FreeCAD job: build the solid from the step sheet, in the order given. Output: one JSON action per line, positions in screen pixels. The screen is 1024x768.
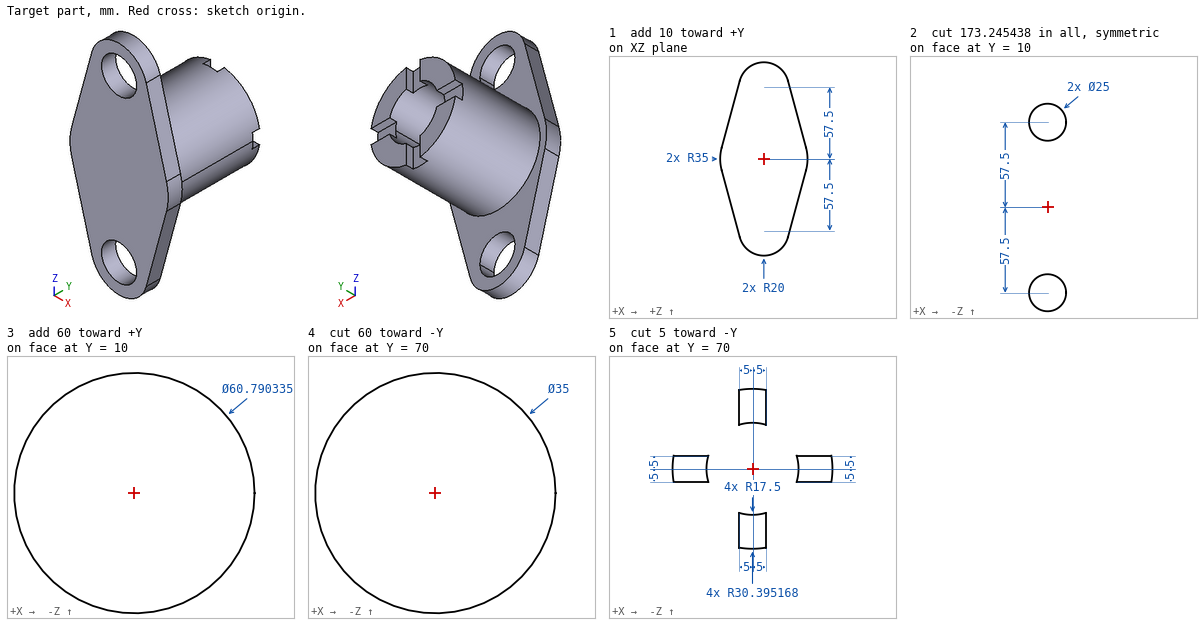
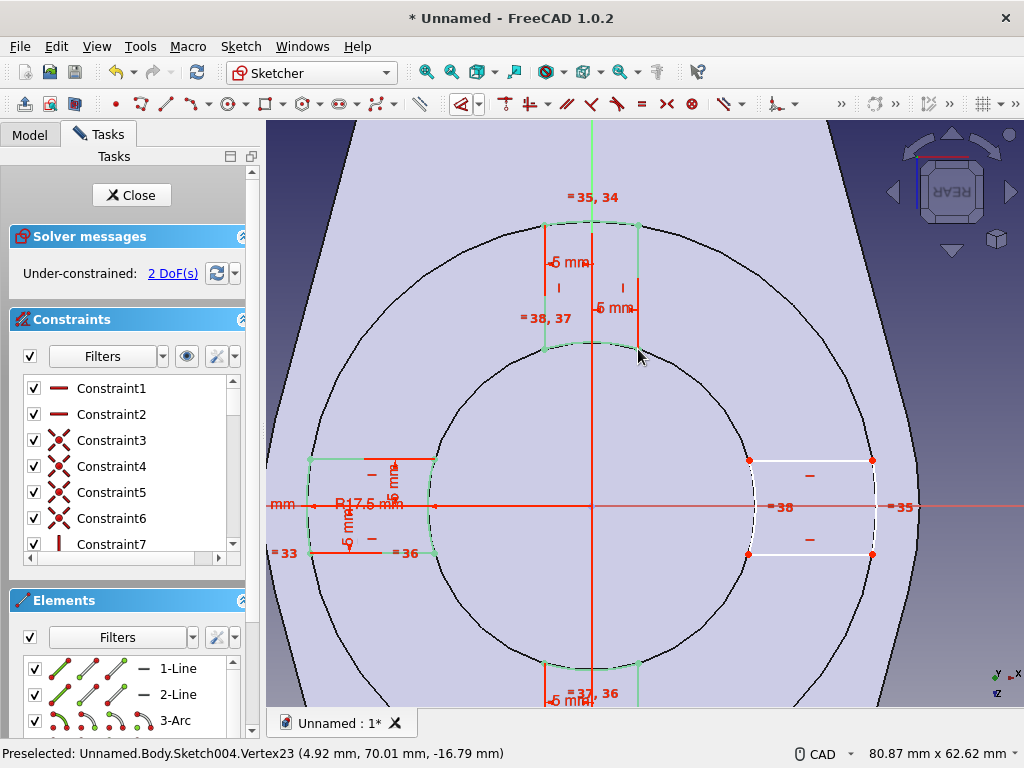
{"action": "scroll", "coordinate": [546, 225], "scroll_direction": "down", "scroll_amount": 2}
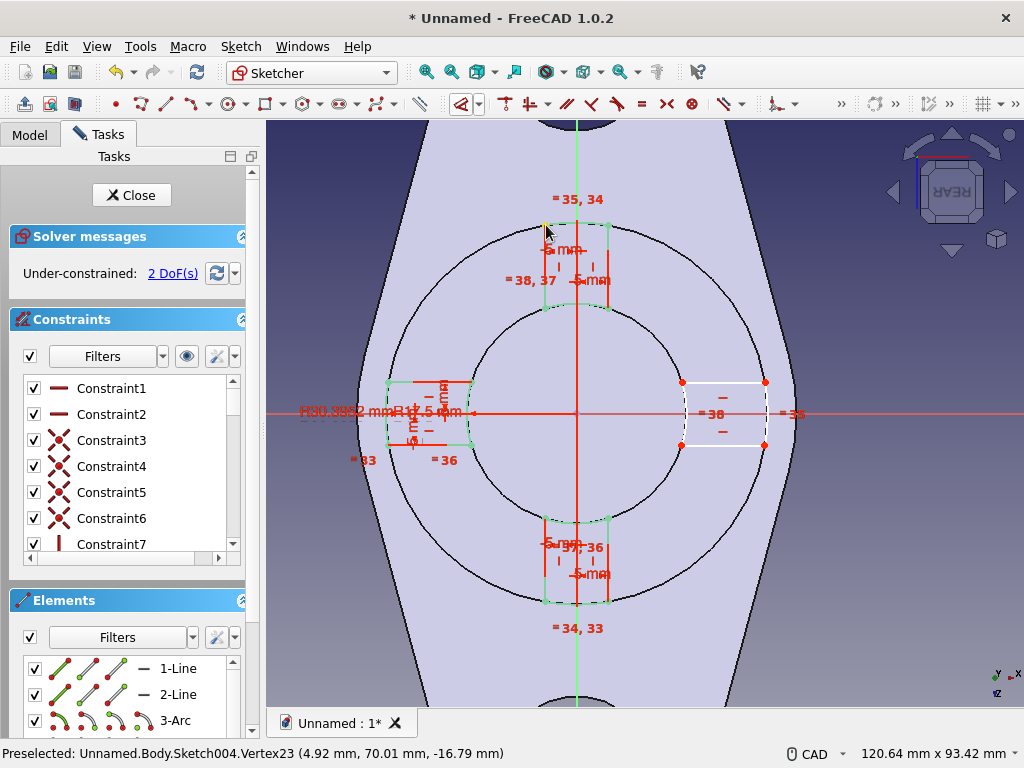
{"action": "scroll", "coordinate": [765, 383], "scroll_direction": "up", "scroll_amount": 2}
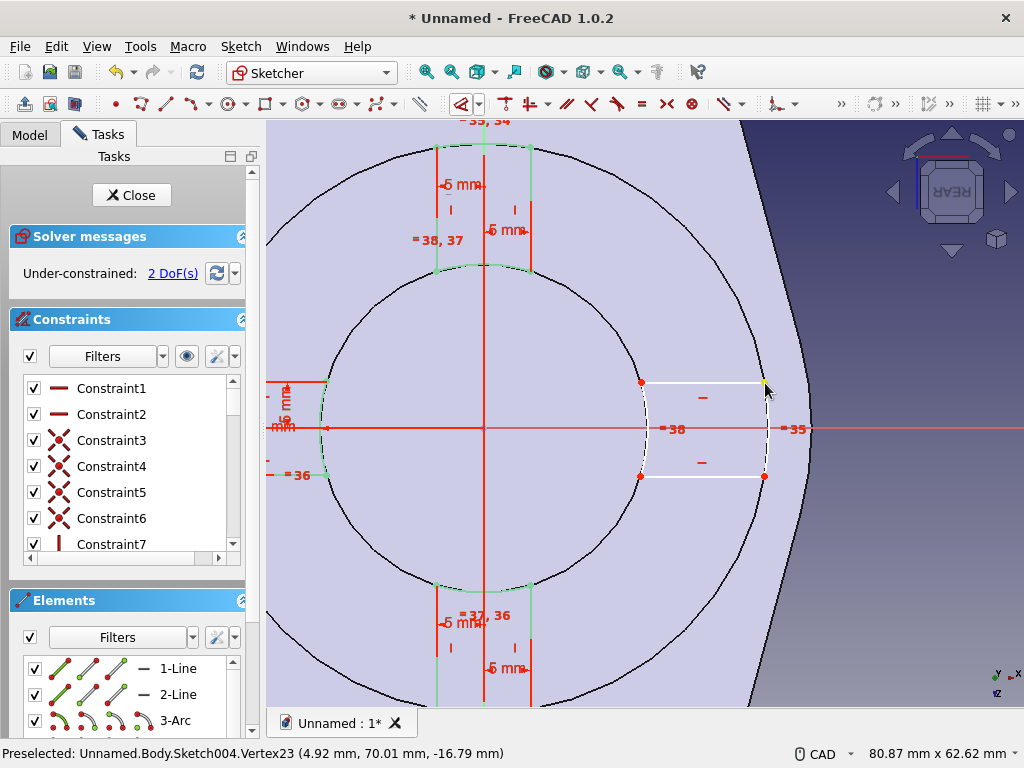
{"action": "left_click", "coordinate": [765, 383]}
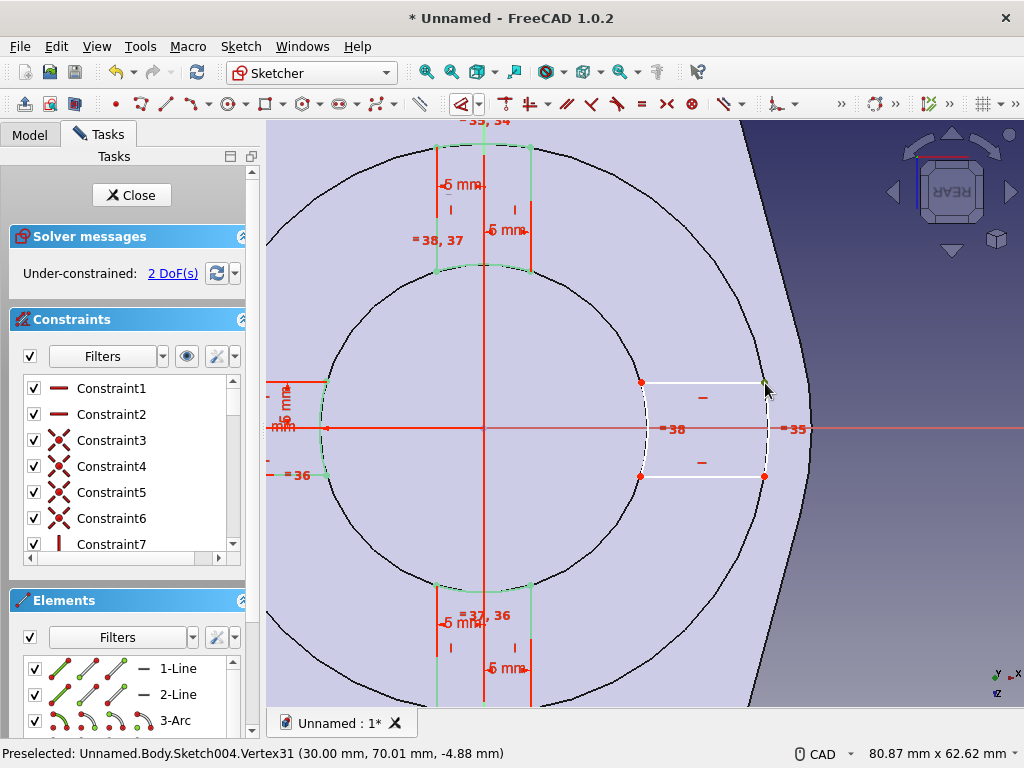
{"action": "key", "text": "i"}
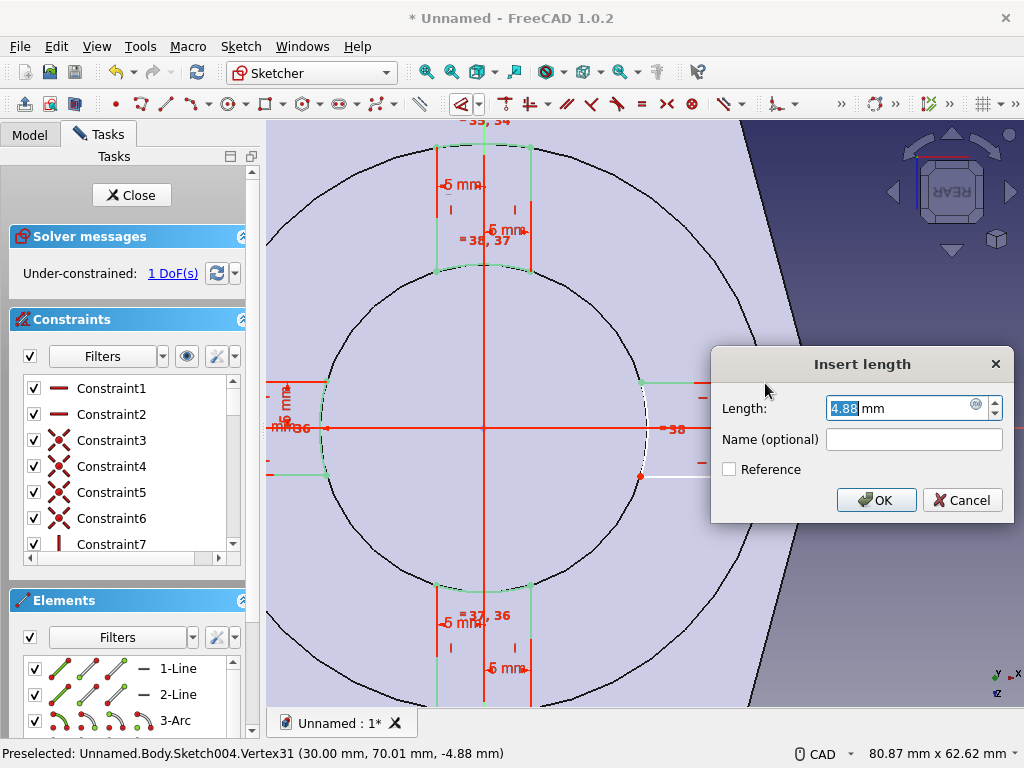
{"action": "type", "text": "5"}
{"action": "key", "text": "Return"}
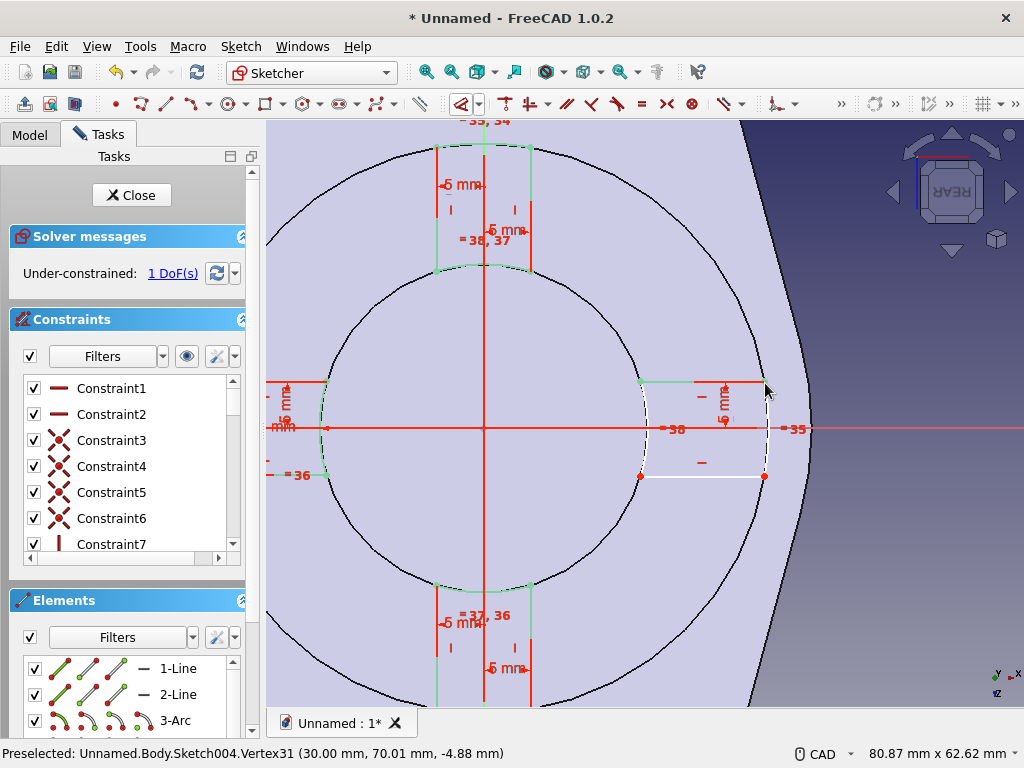
{"action": "left_click", "coordinate": [641, 477]}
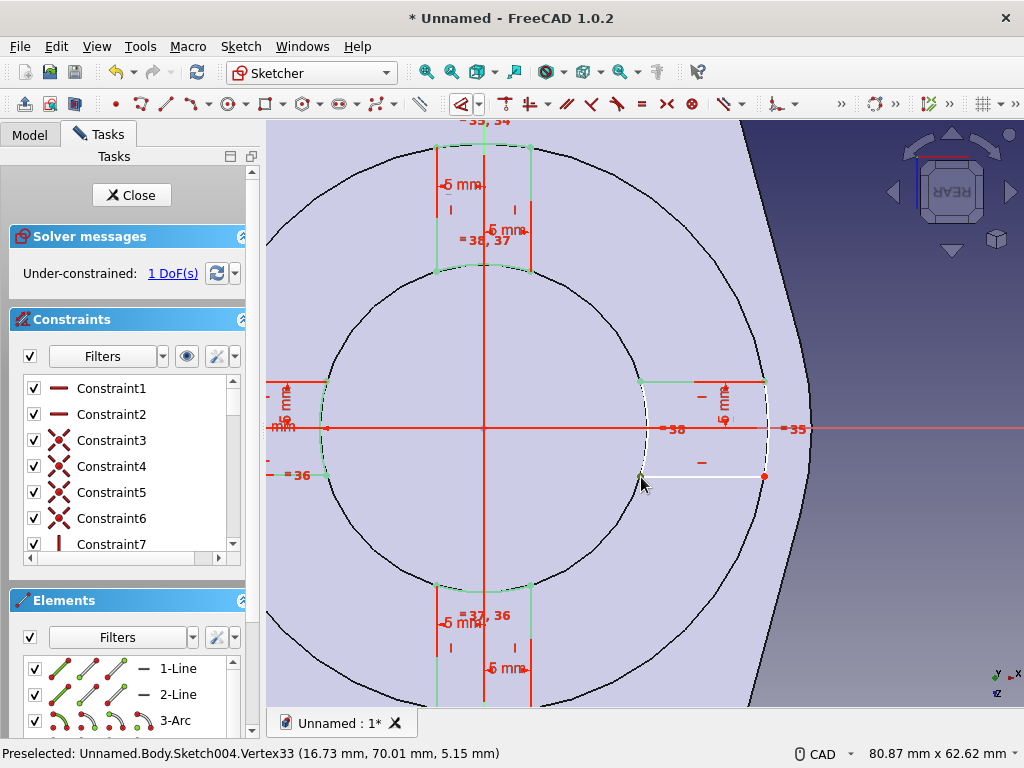
{"action": "left_click", "coordinate": [478, 104]}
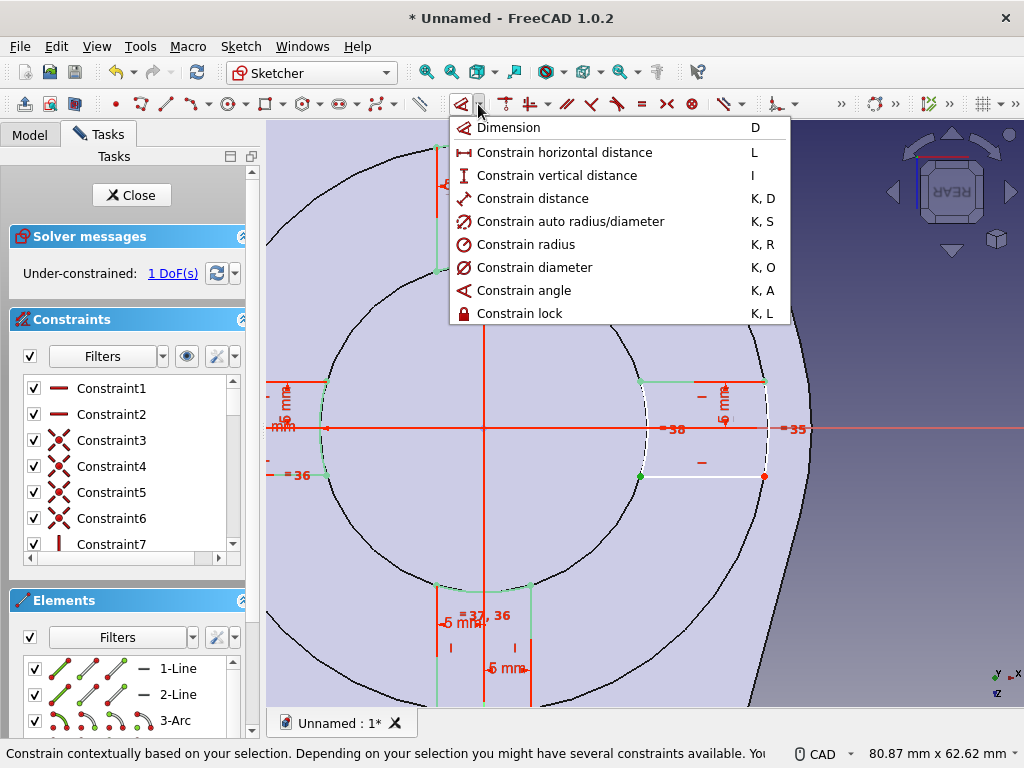
{"action": "left_click", "coordinate": [620, 176]}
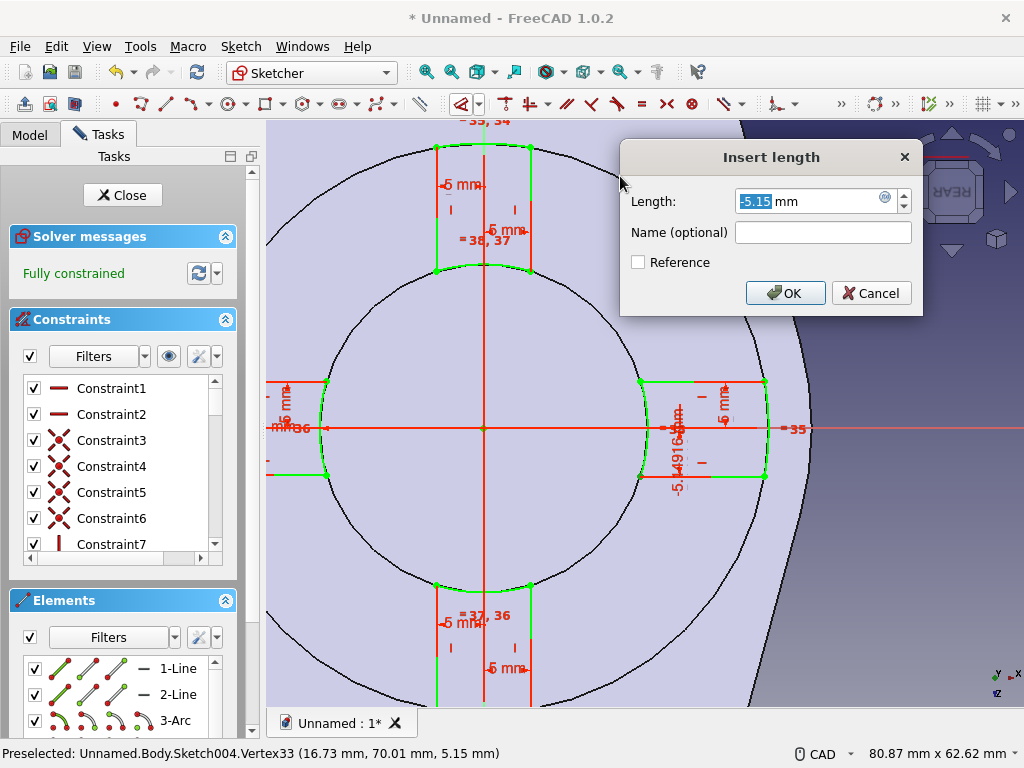
{"action": "type", "text": "-5"}
{"action": "key", "text": "Return"}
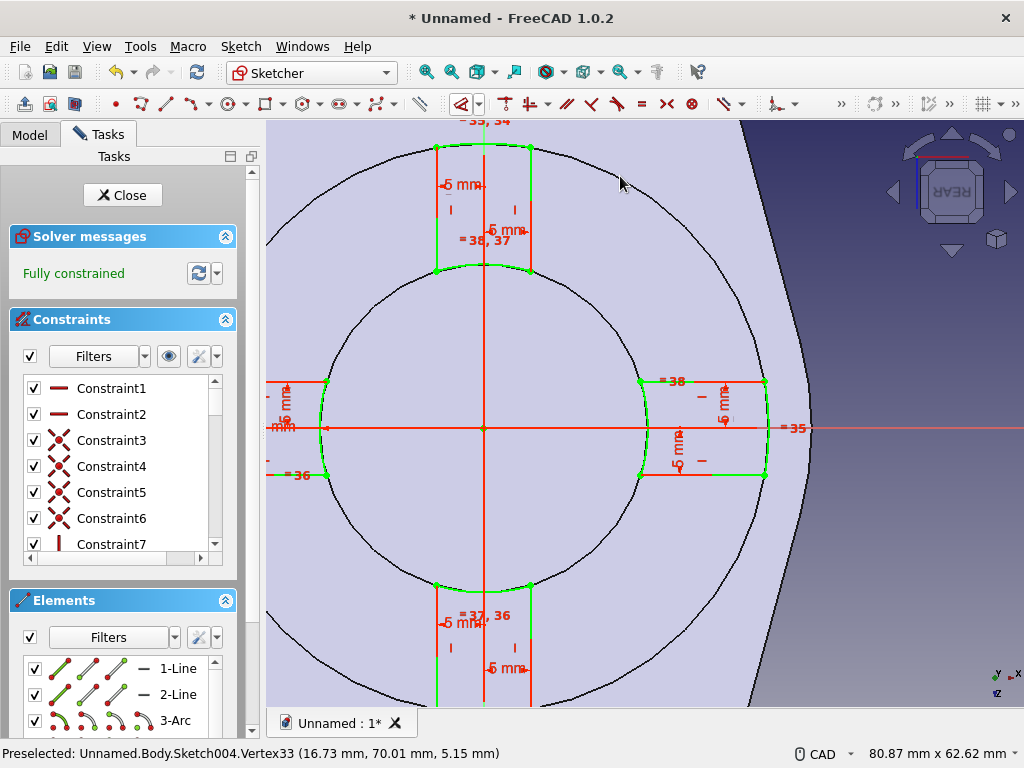
{"action": "left_click", "coordinate": [123, 195]}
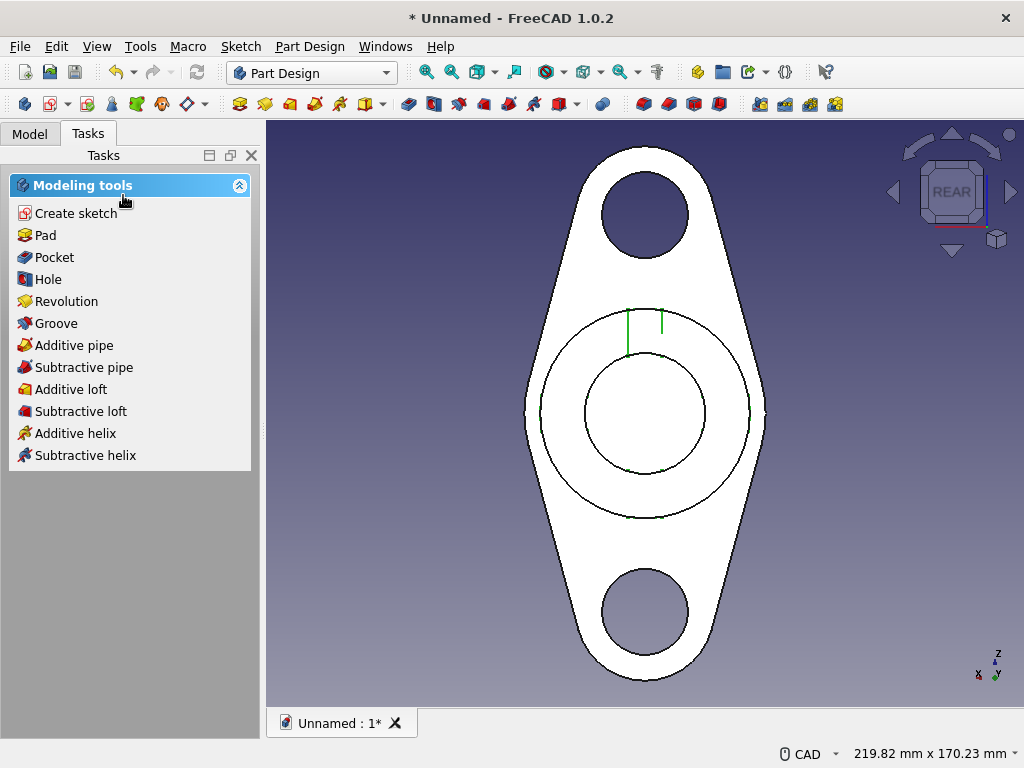
{"action": "left_click", "coordinate": [409, 104]}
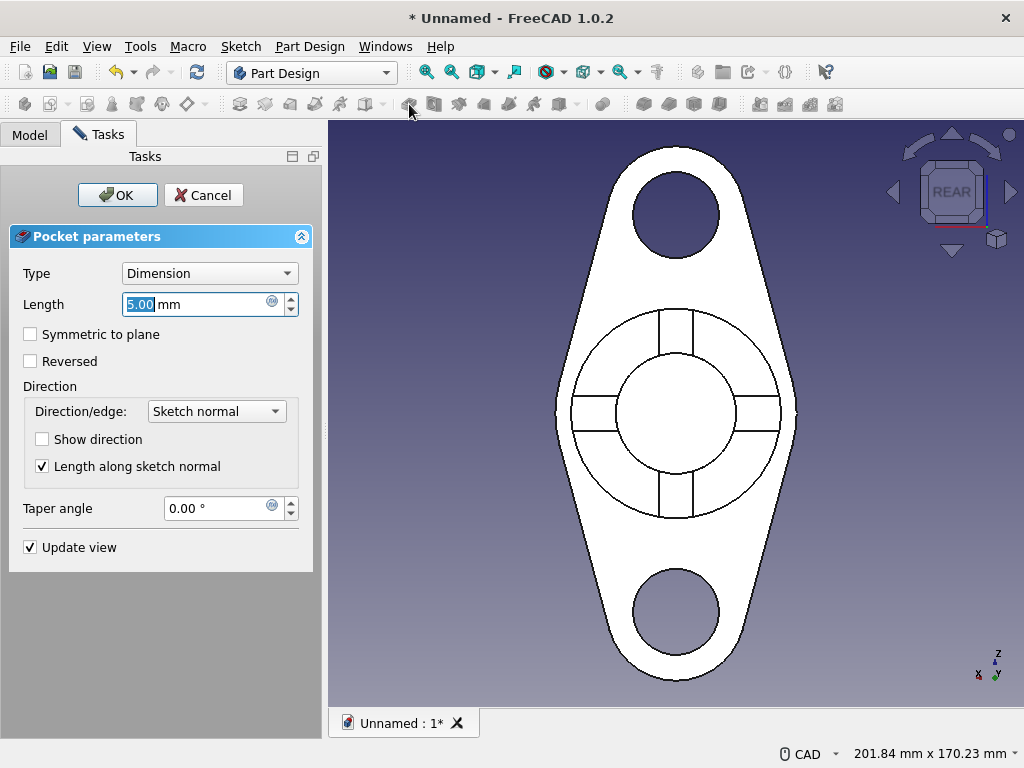
{"action": "type", "text": "5"}
{"action": "key", "text": "Tab"}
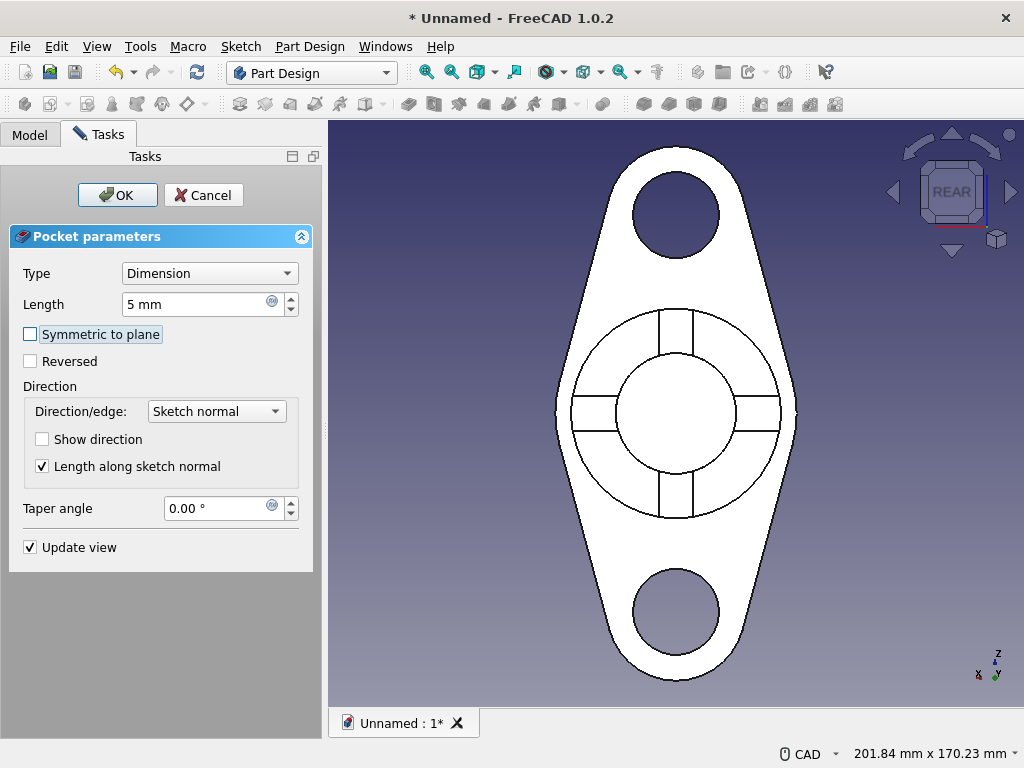
{"action": "left_click", "coordinate": [118, 195]}